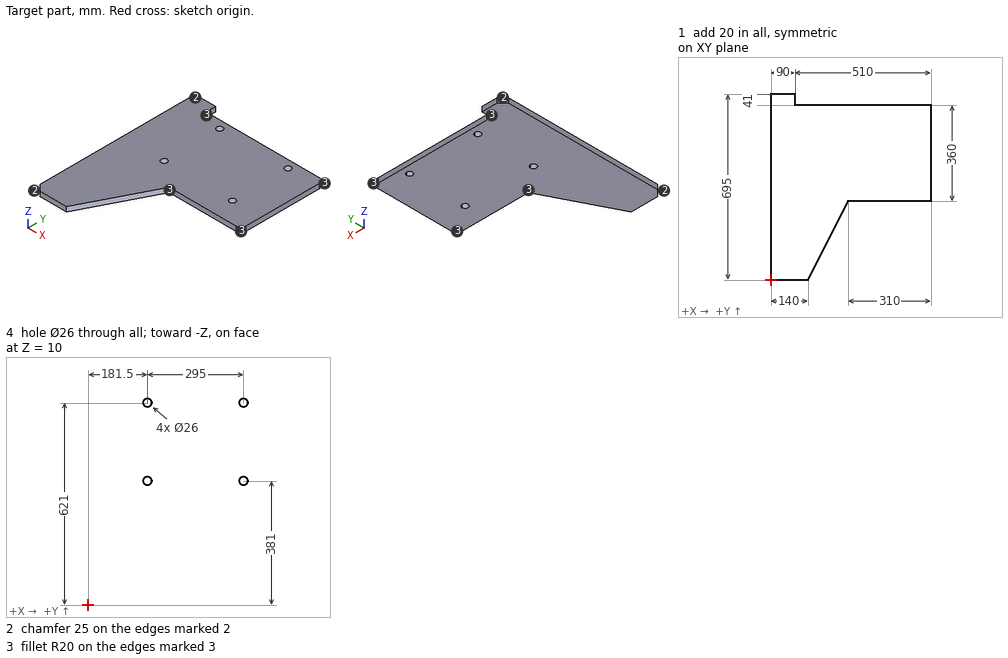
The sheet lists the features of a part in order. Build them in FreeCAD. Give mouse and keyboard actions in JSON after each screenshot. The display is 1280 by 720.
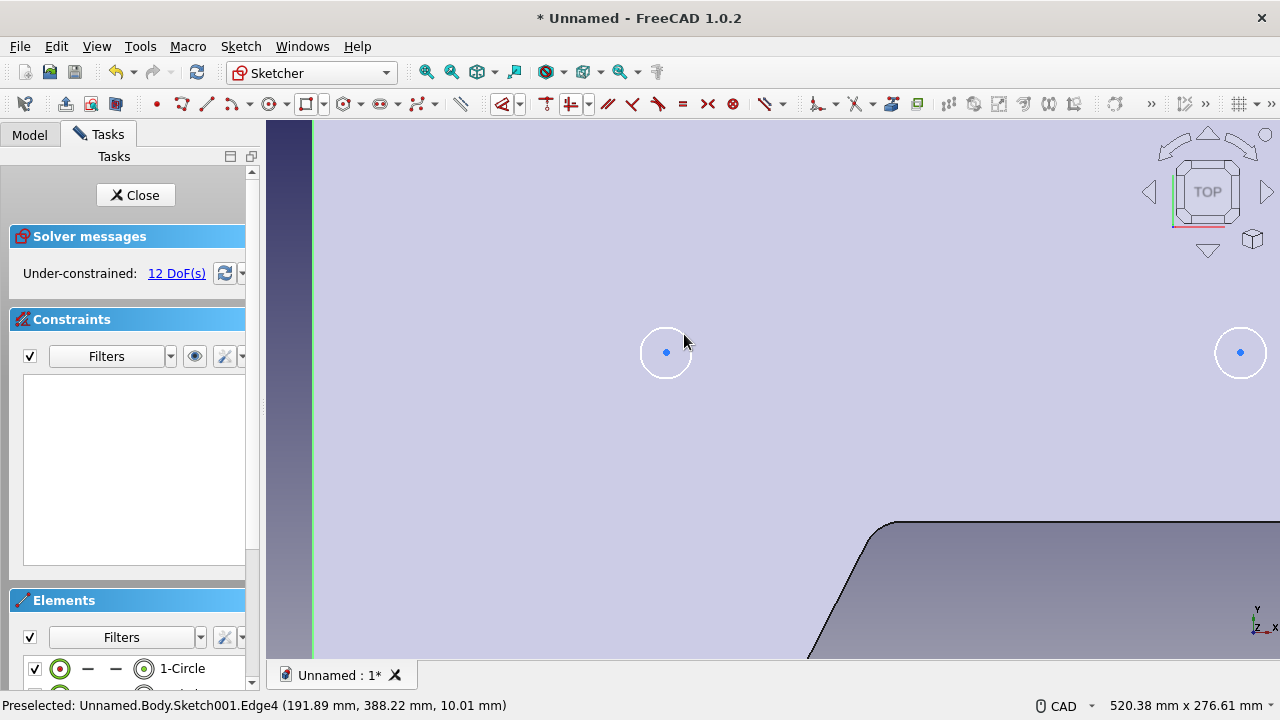
{"action": "scroll", "coordinate": [668, 352], "scroll_direction": "down", "scroll_amount": 6}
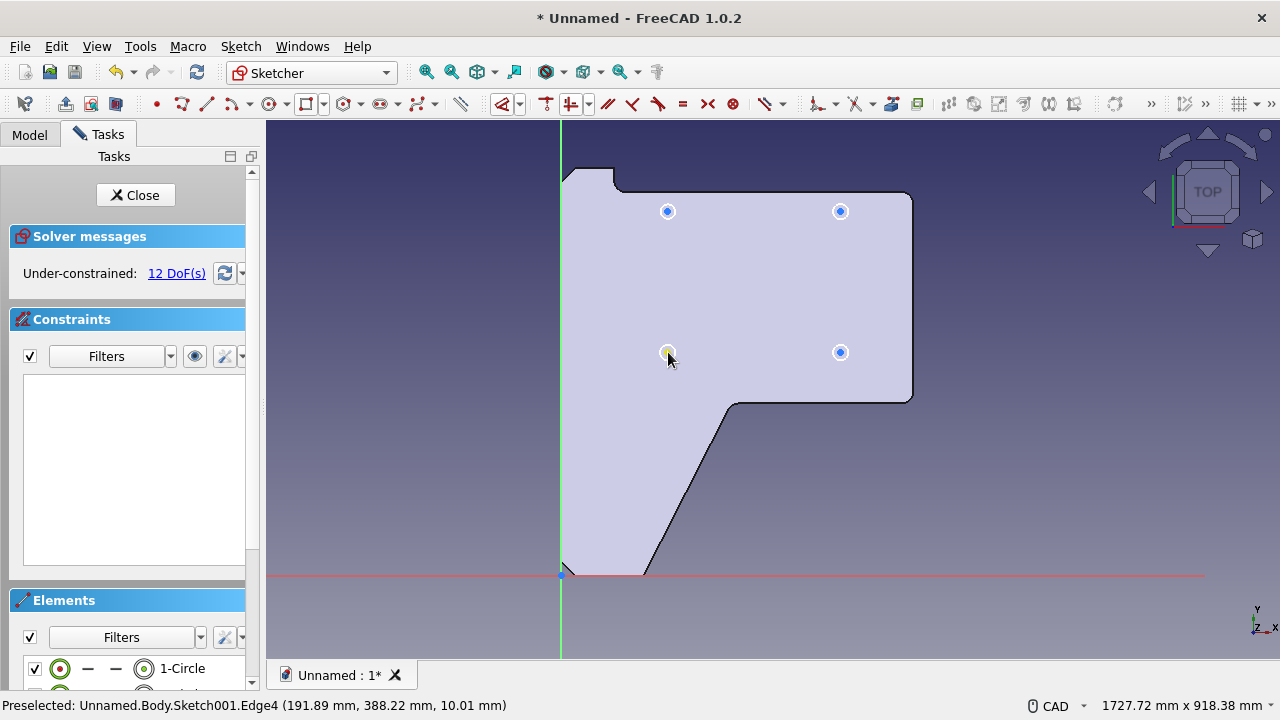
{"action": "scroll", "coordinate": [673, 207], "scroll_direction": "up", "scroll_amount": 4}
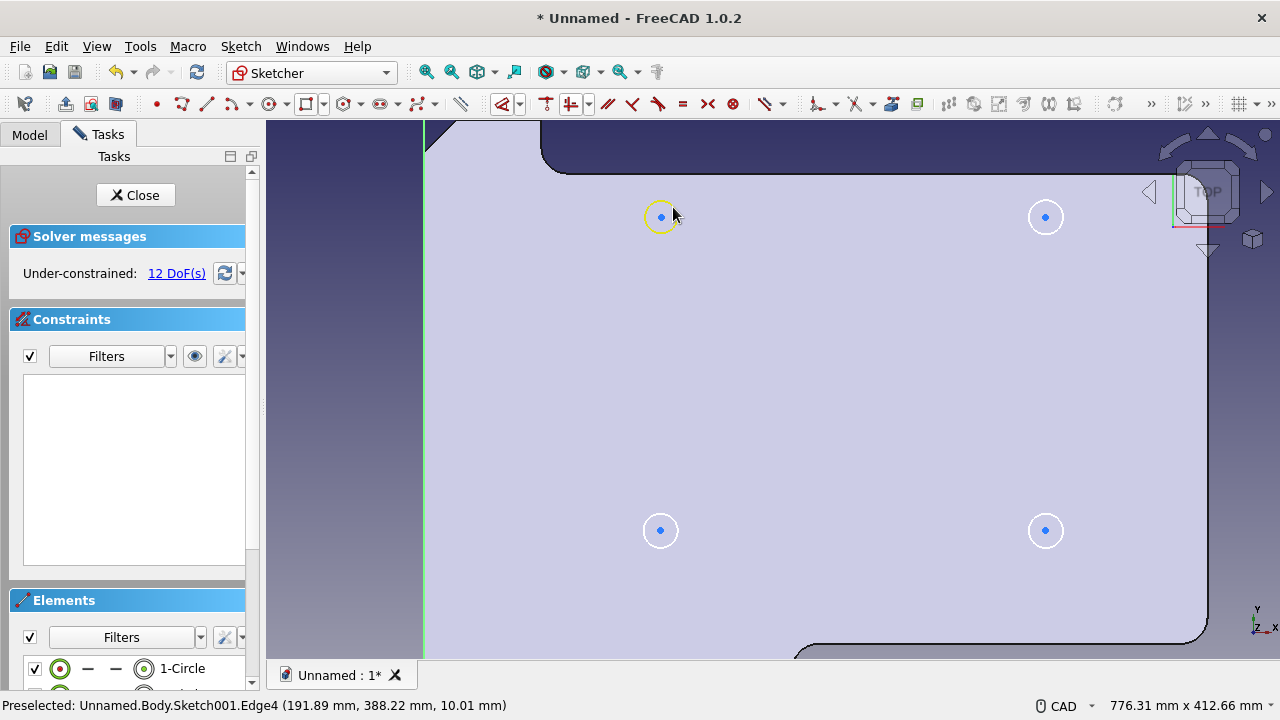
{"action": "left_click", "coordinate": [673, 206]}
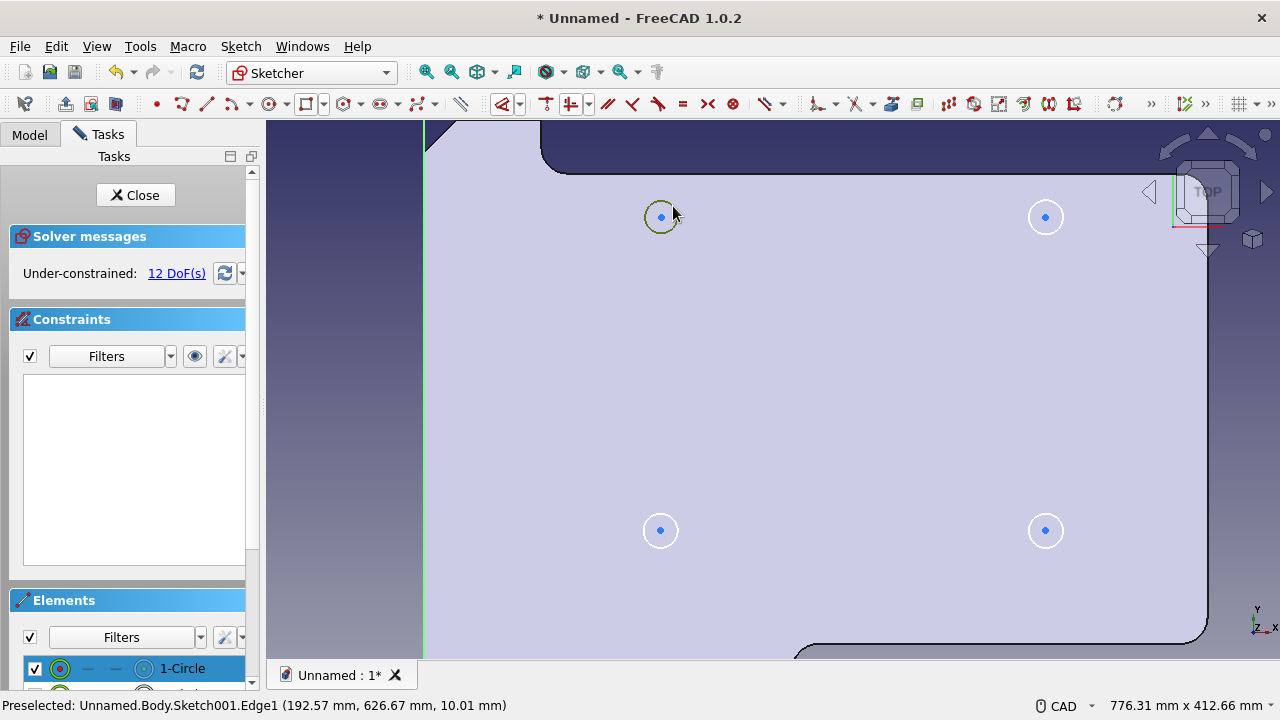
{"action": "left_click", "coordinate": [1058, 205]}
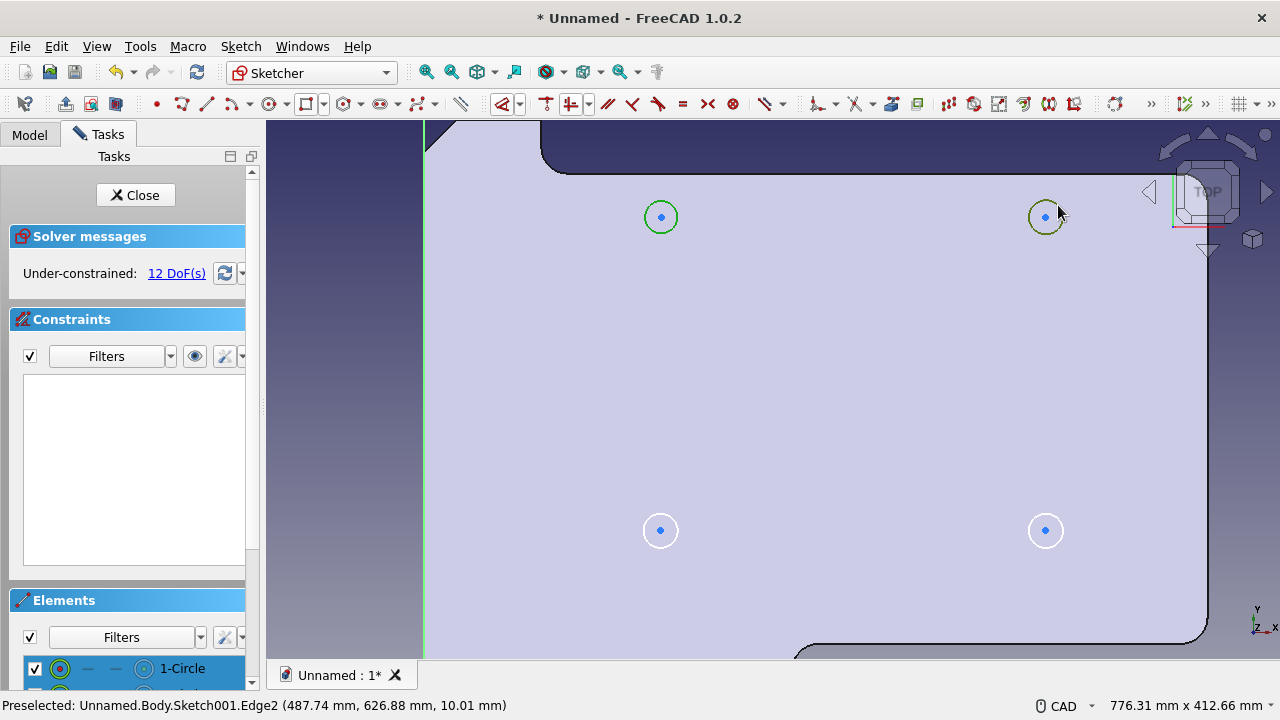
{"action": "left_click", "coordinate": [1058, 519]}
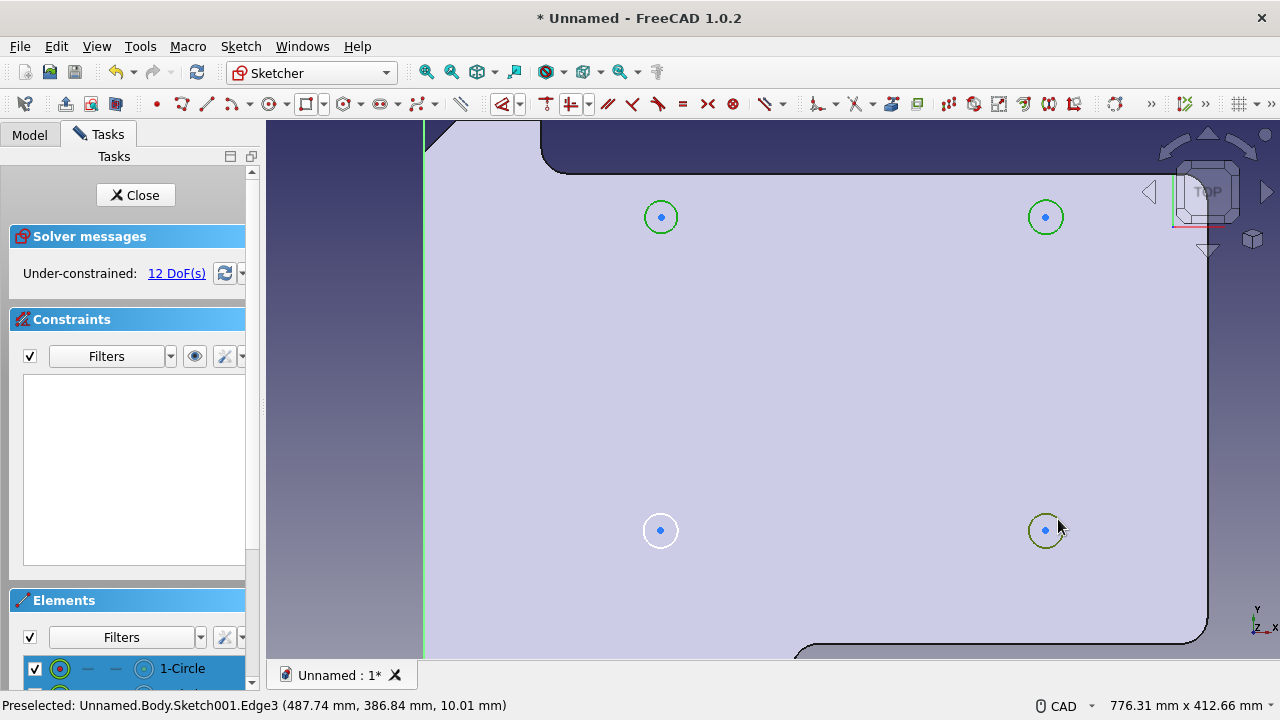
{"action": "left_click", "coordinate": [673, 519]}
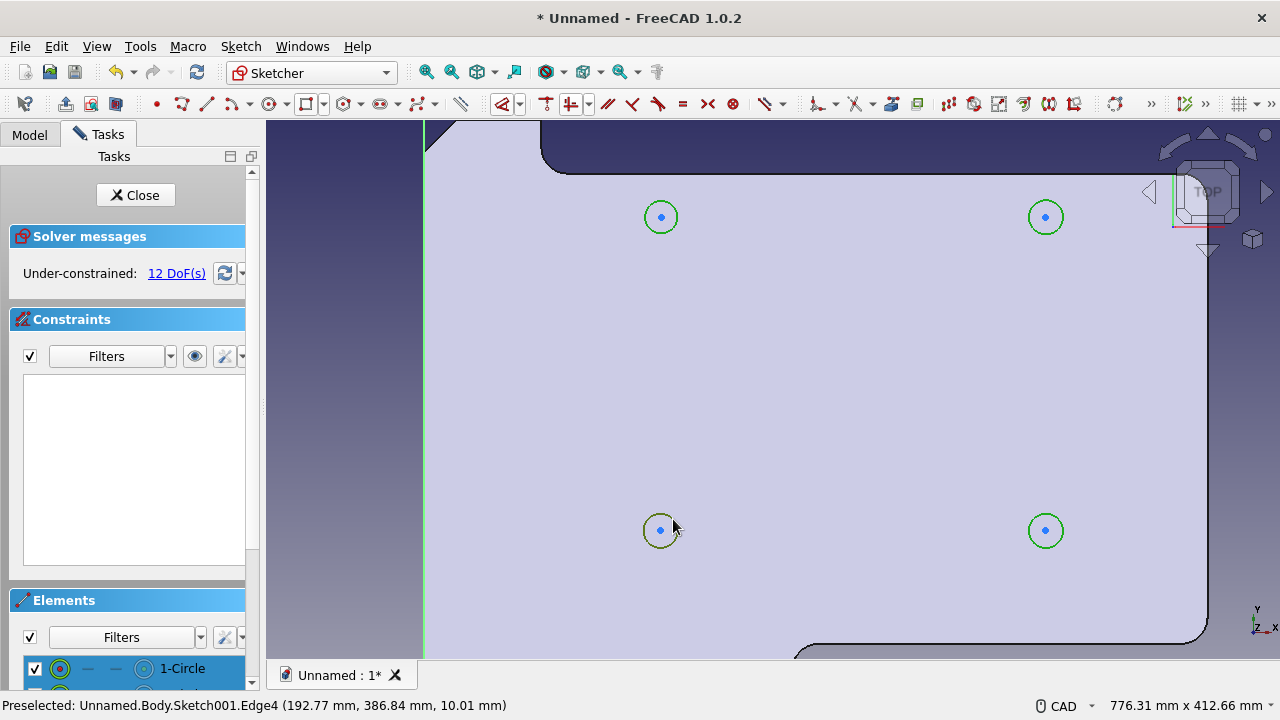
{"action": "left_click", "coordinate": [683, 104]}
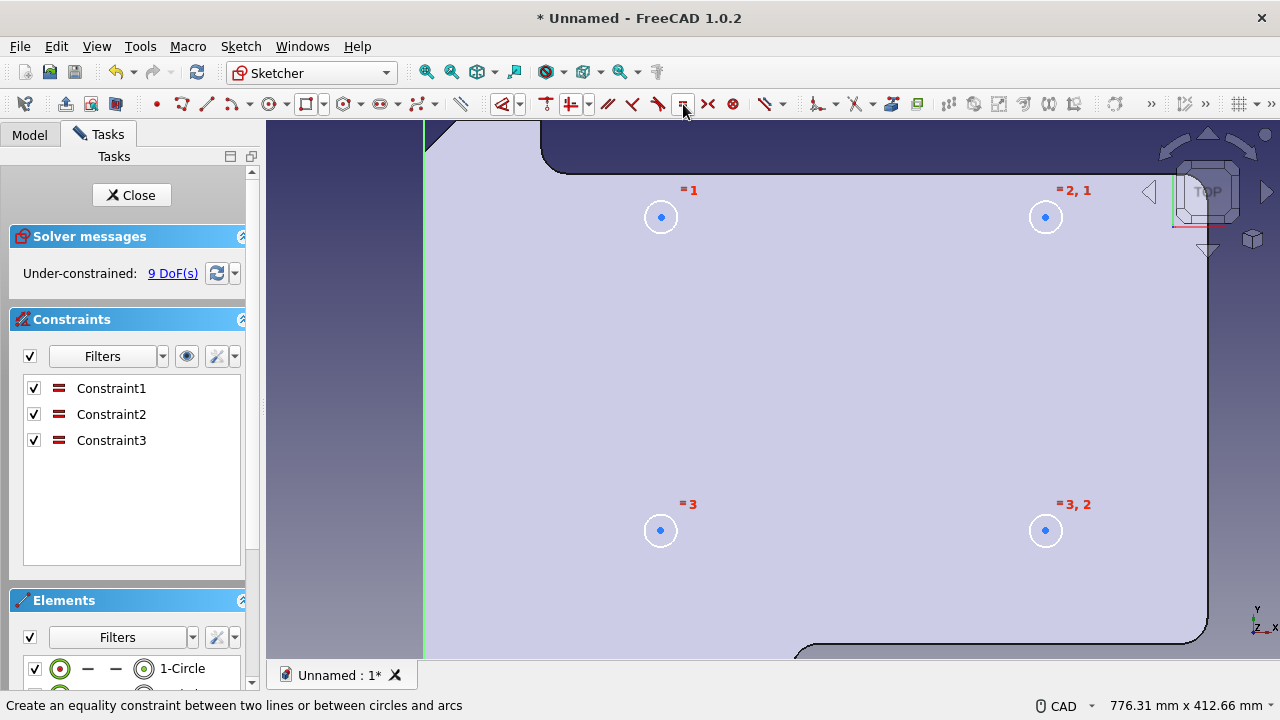
{"action": "left_click", "coordinate": [661, 217]}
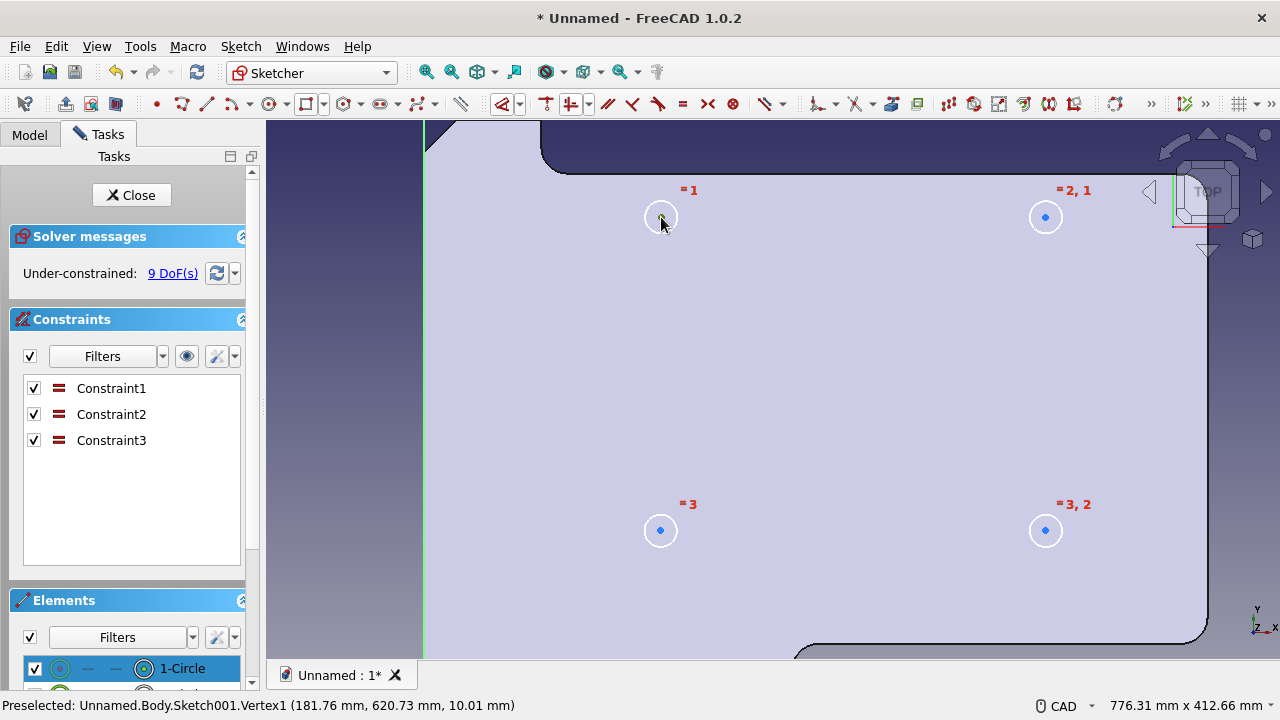
{"action": "left_click", "coordinate": [1046, 217]}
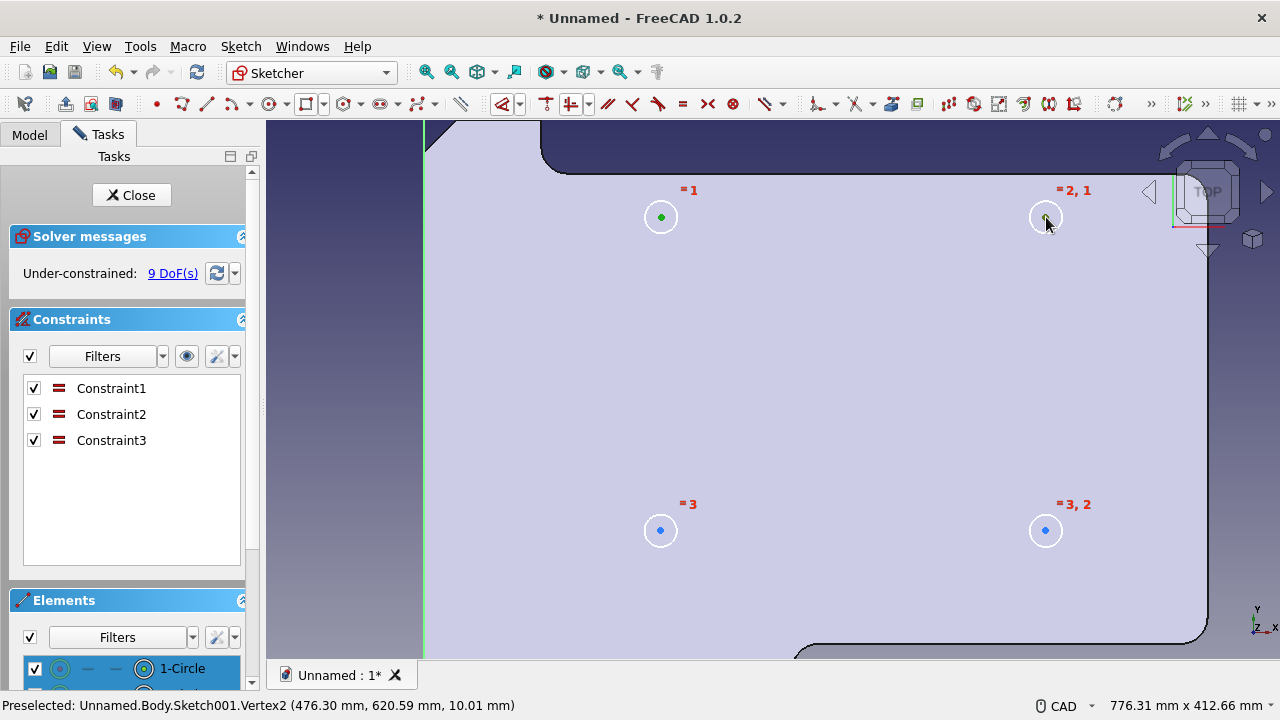
{"action": "left_click", "coordinate": [588, 104]}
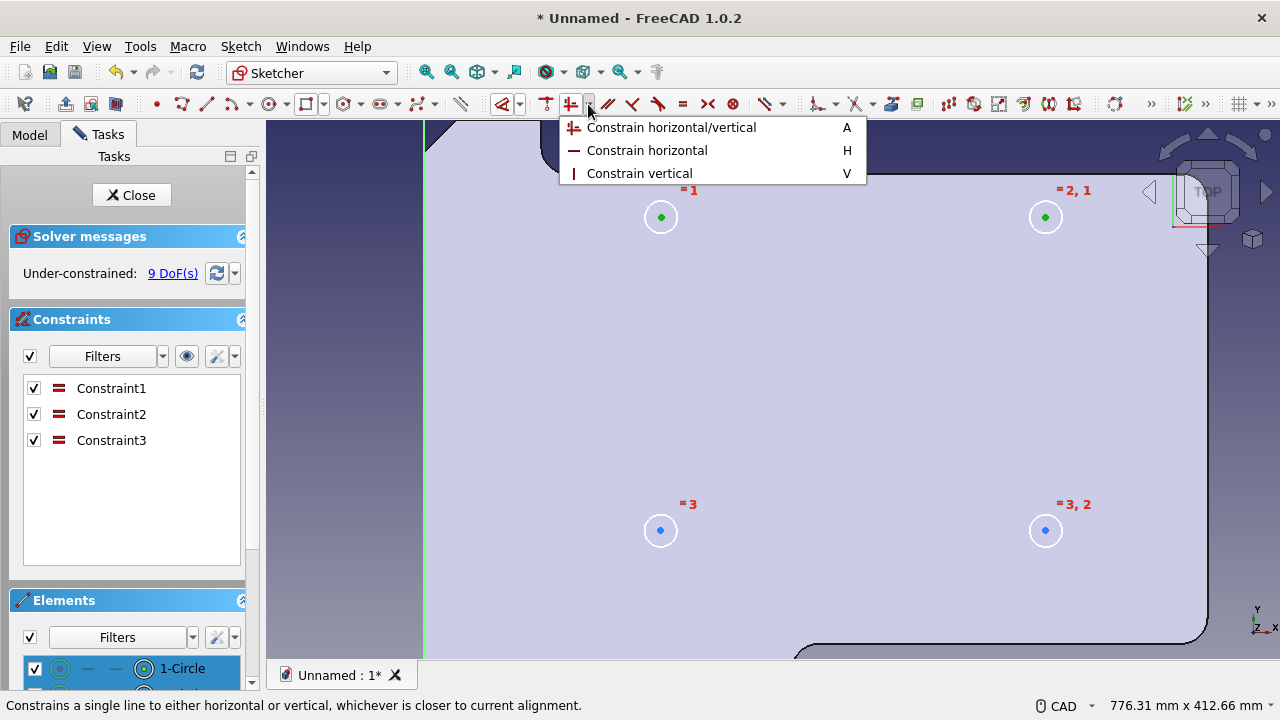
{"action": "left_click", "coordinate": [713, 150]}